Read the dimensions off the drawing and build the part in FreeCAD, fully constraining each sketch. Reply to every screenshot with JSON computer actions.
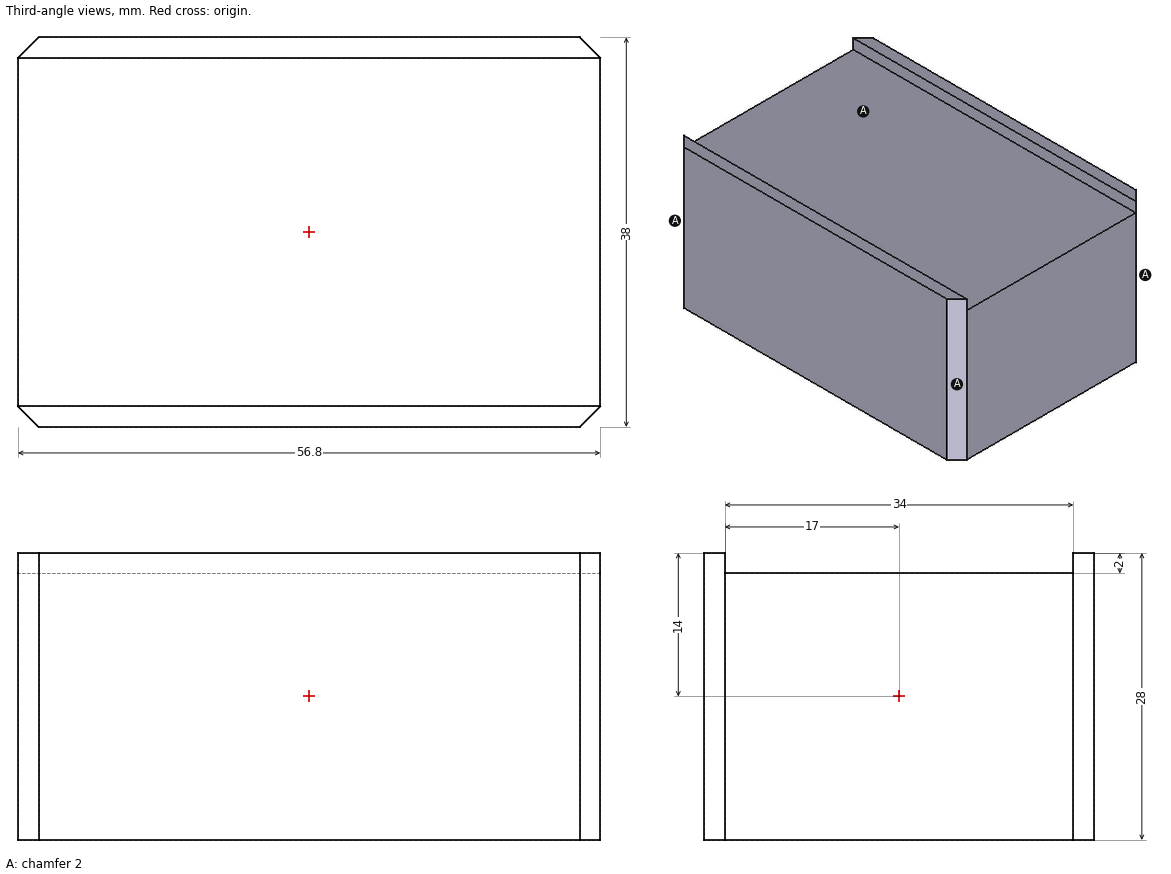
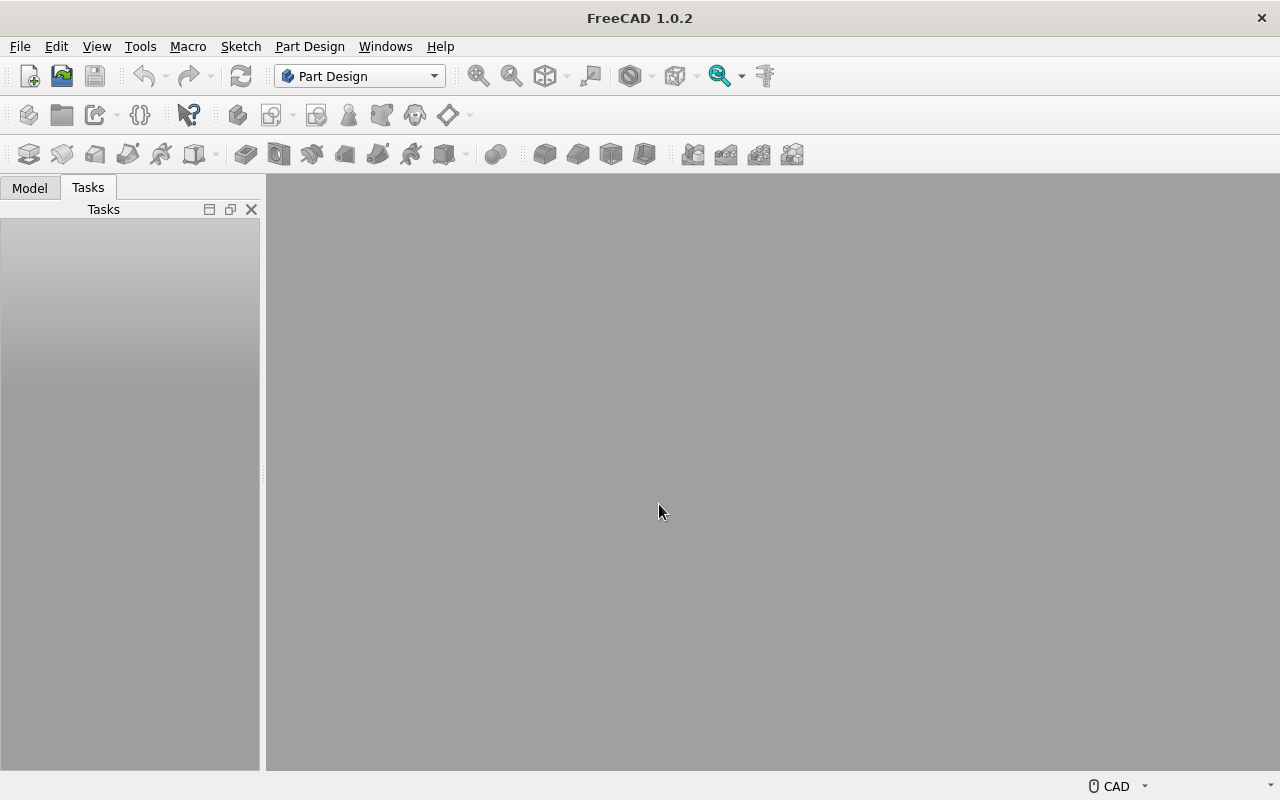
{"action": "left_click", "coordinate": [29, 76]}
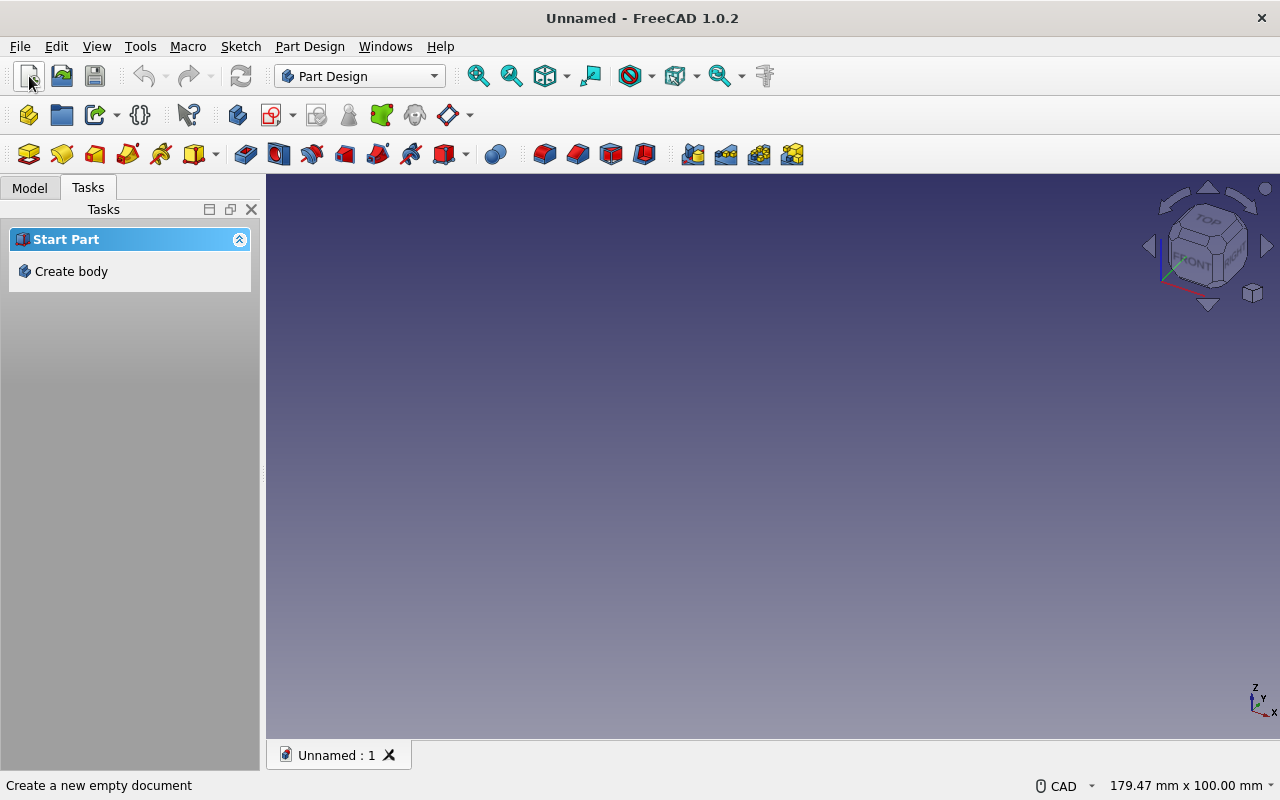
{"action": "left_click", "coordinate": [270, 116]}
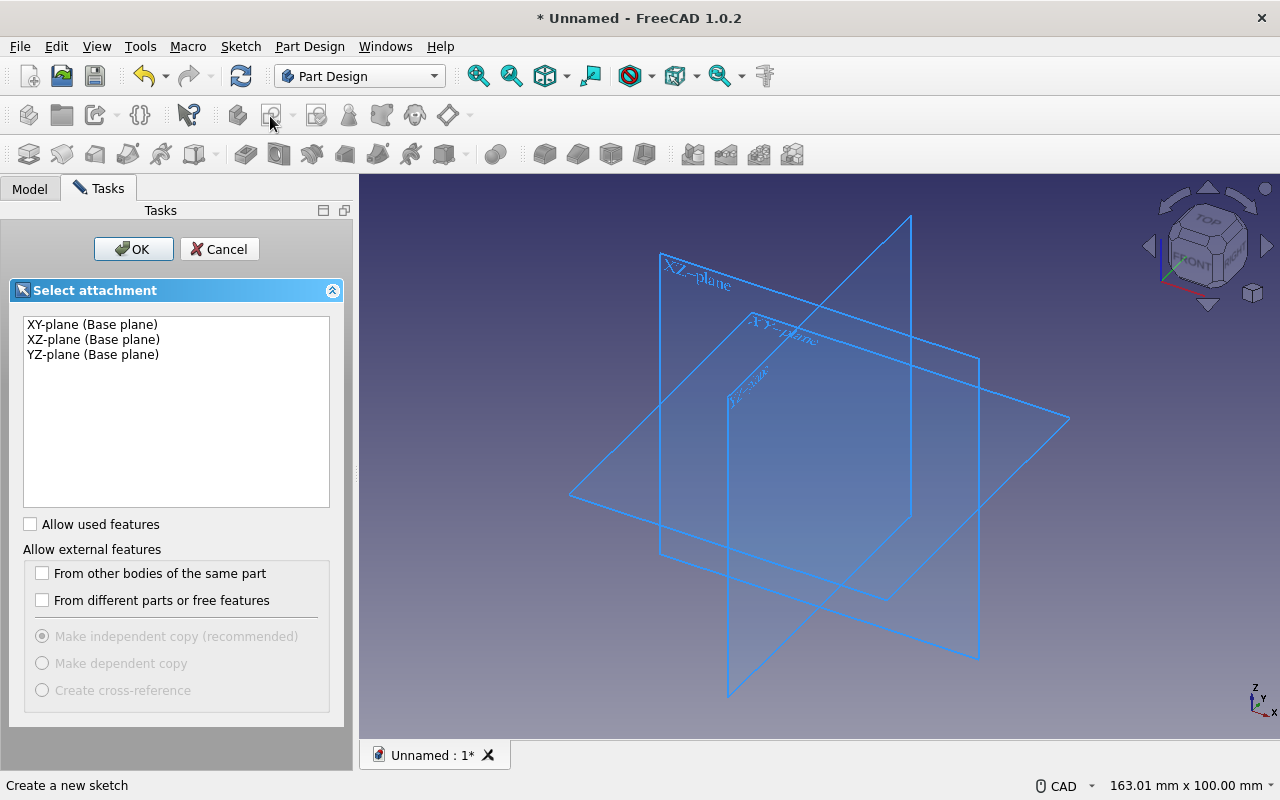
{"action": "left_click", "coordinate": [84, 324]}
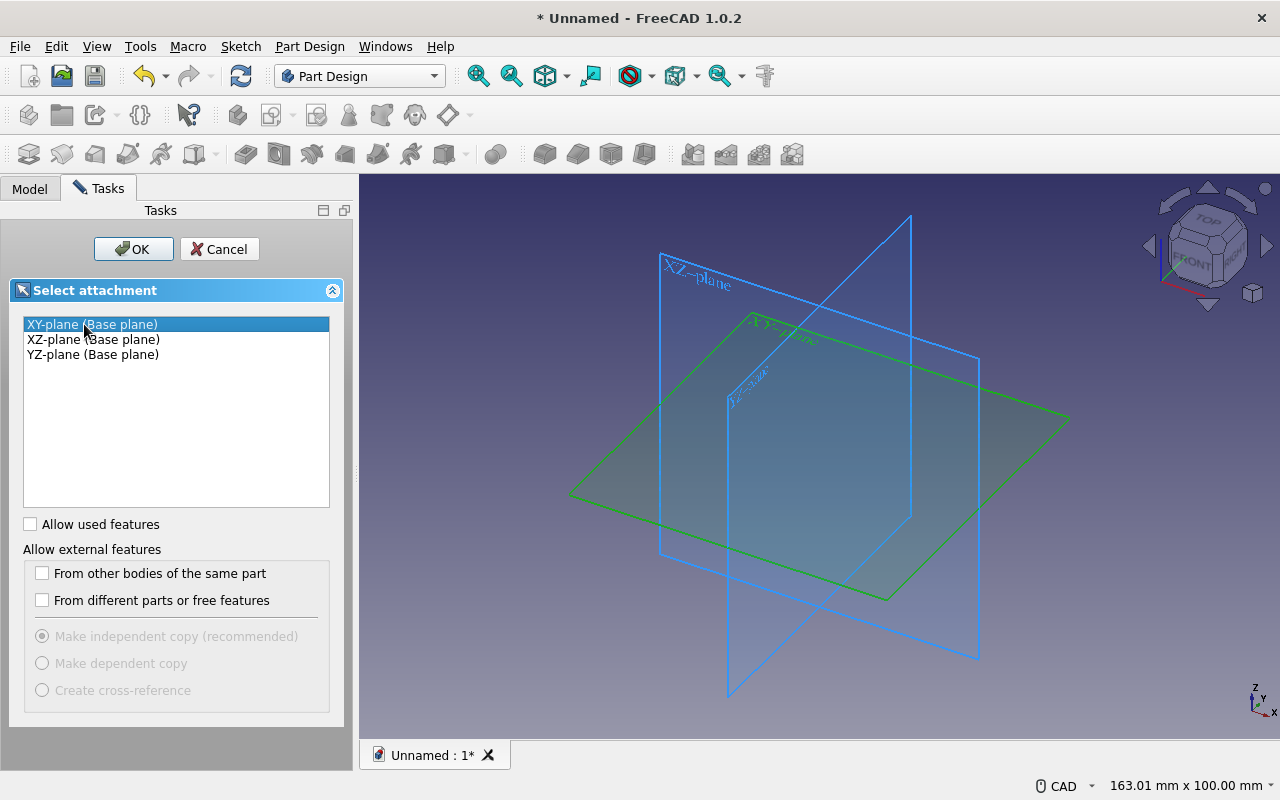
{"action": "left_click", "coordinate": [134, 249]}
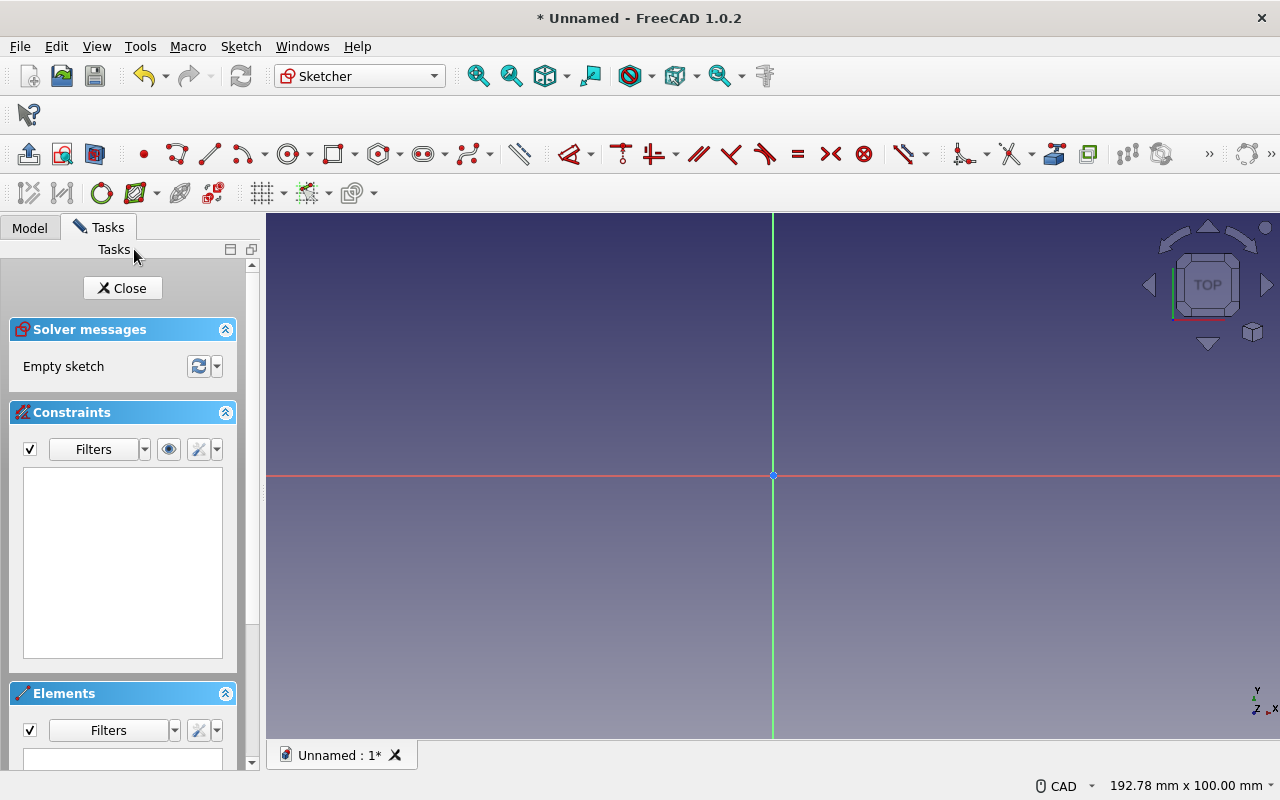
{"action": "scroll", "coordinate": [856, 476], "scroll_direction": "up", "scroll_amount": 3}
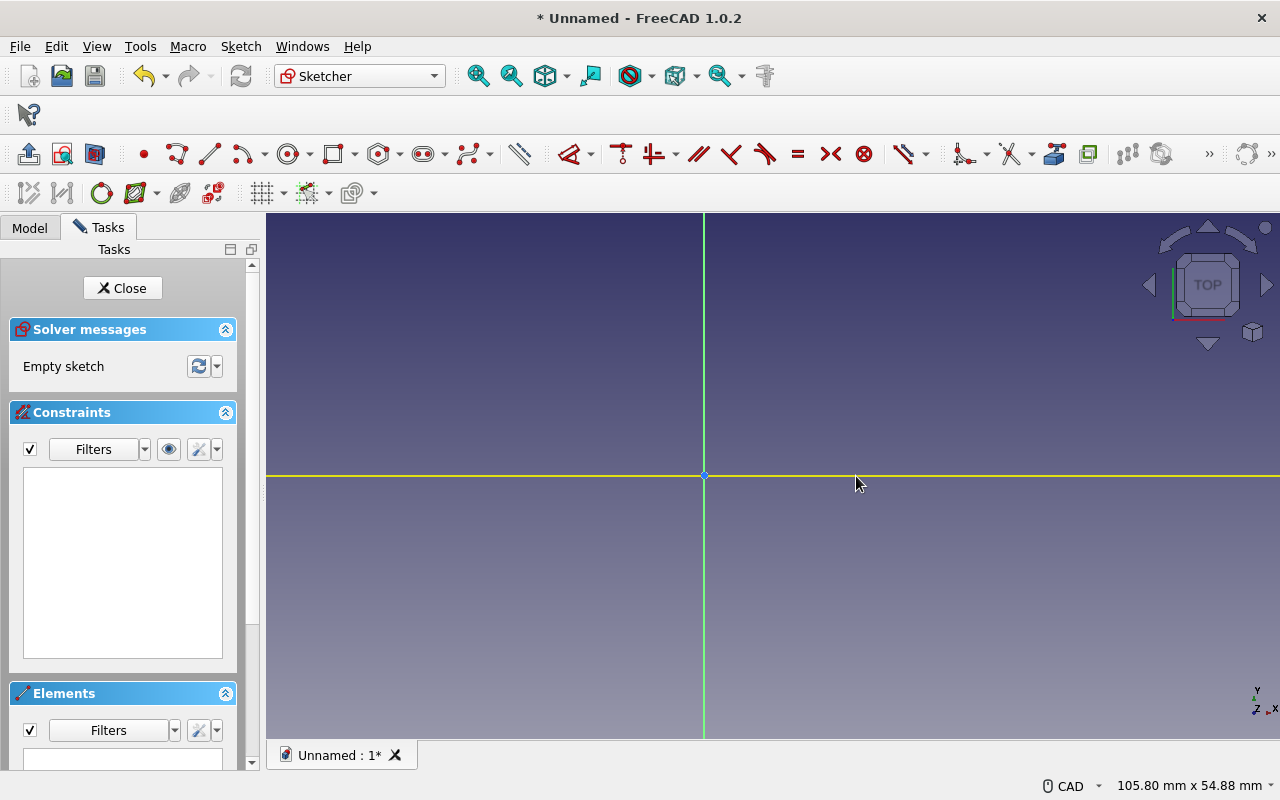
{"action": "left_click", "coordinate": [354, 154]}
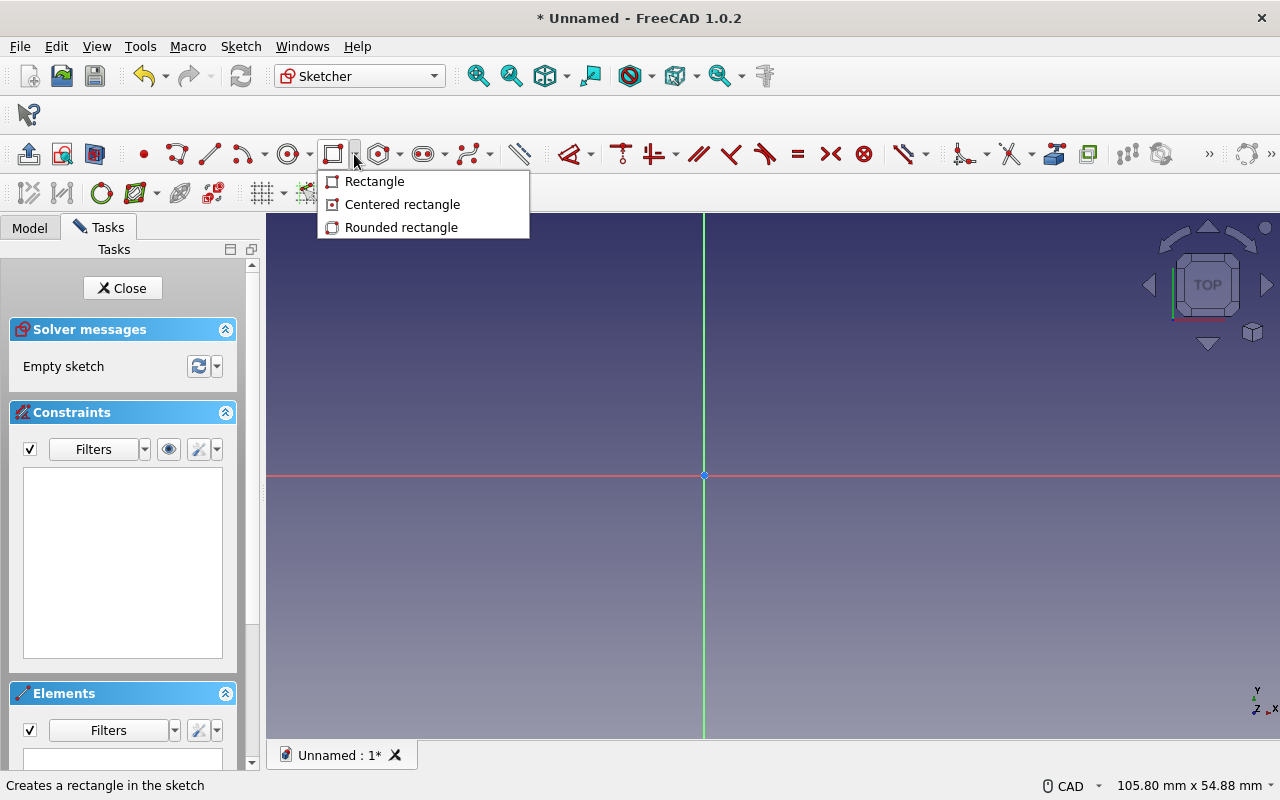
{"action": "left_click", "coordinate": [424, 204]}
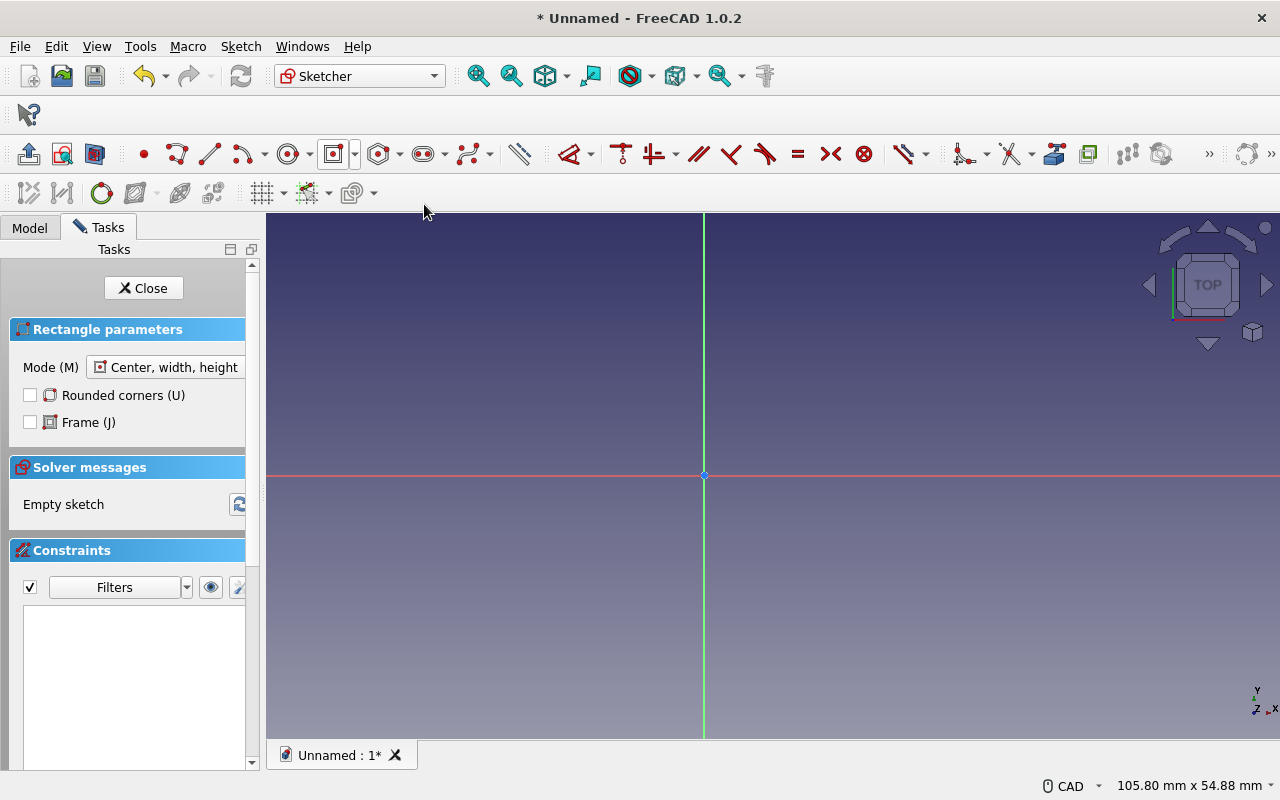
{"action": "left_click", "coordinate": [704, 476]}
{"action": "mouse_move", "coordinate": [976, 293]}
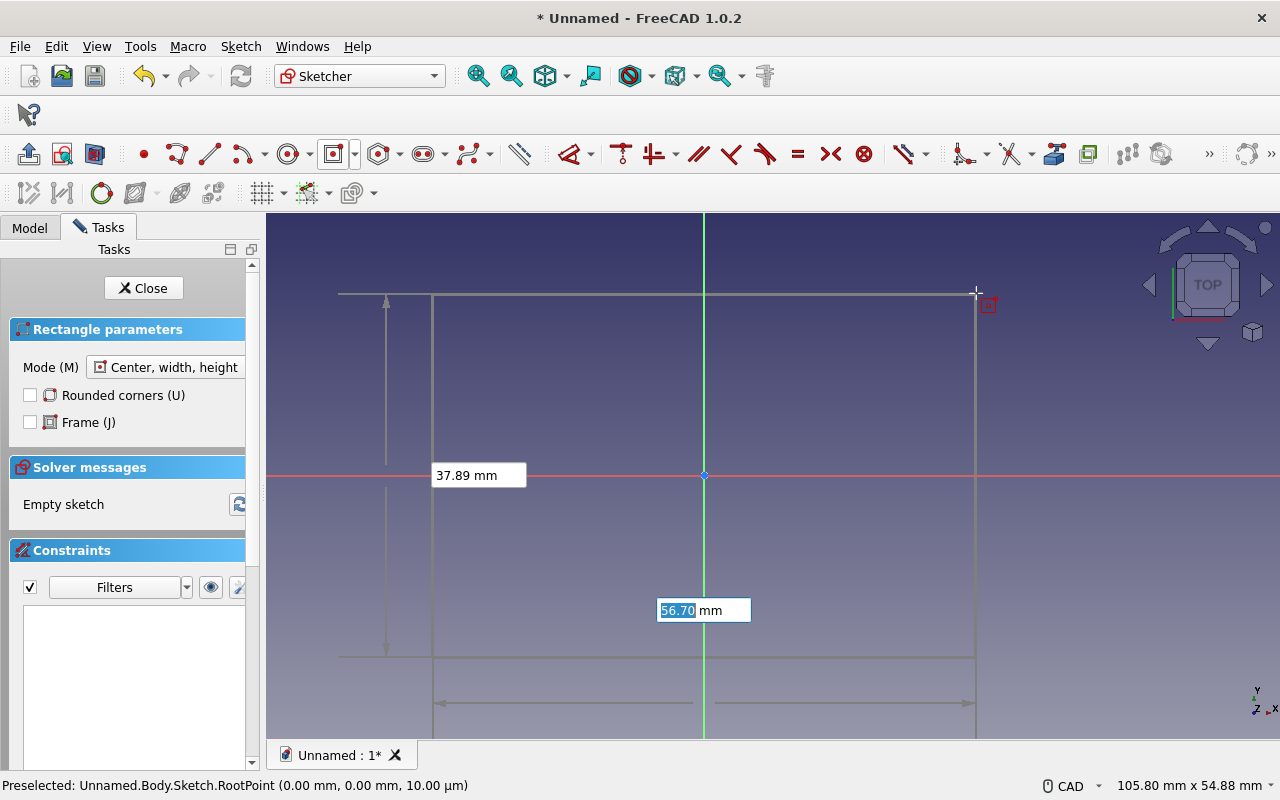
{"action": "type", "text": "56.8"}
{"action": "key", "text": "Tab"}
{"action": "type", "text": "38"}
{"action": "key", "text": "Return"}
{"action": "key", "text": "Escape"}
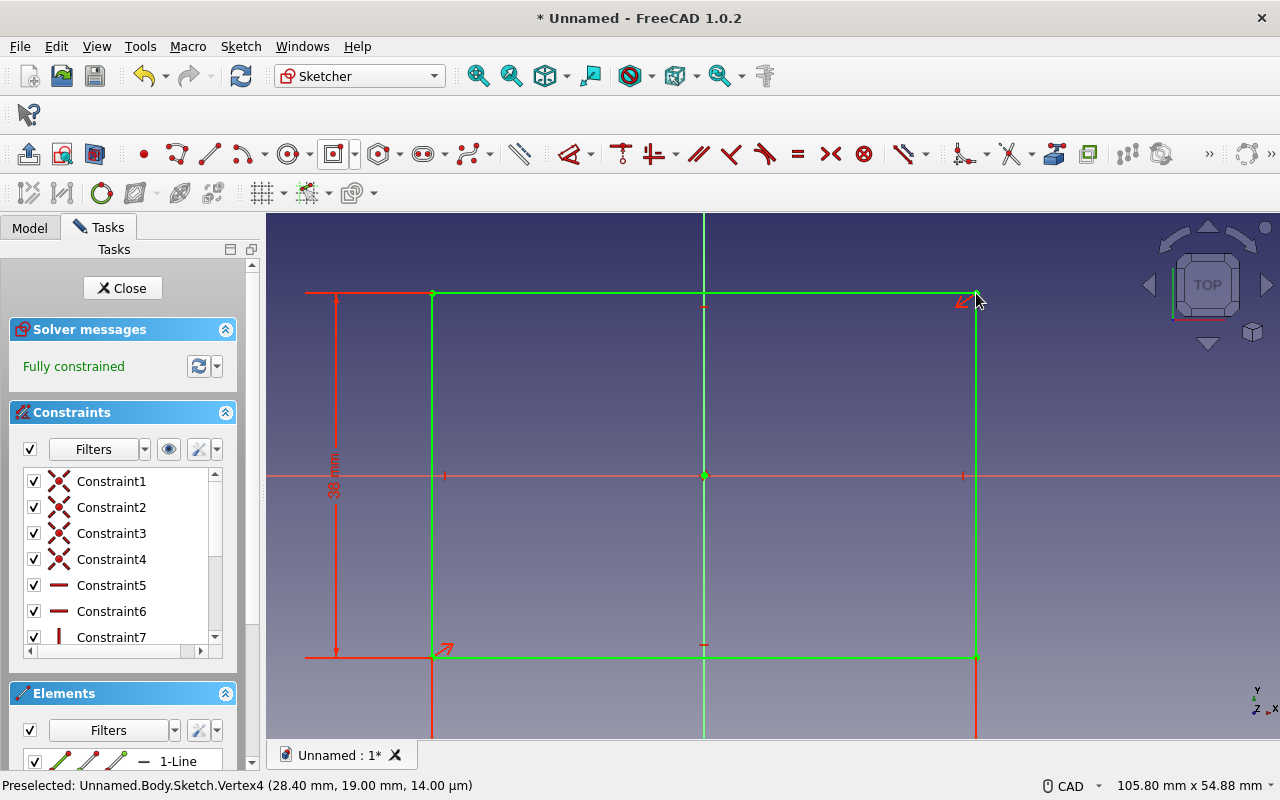
{"action": "left_click", "coordinate": [123, 288]}